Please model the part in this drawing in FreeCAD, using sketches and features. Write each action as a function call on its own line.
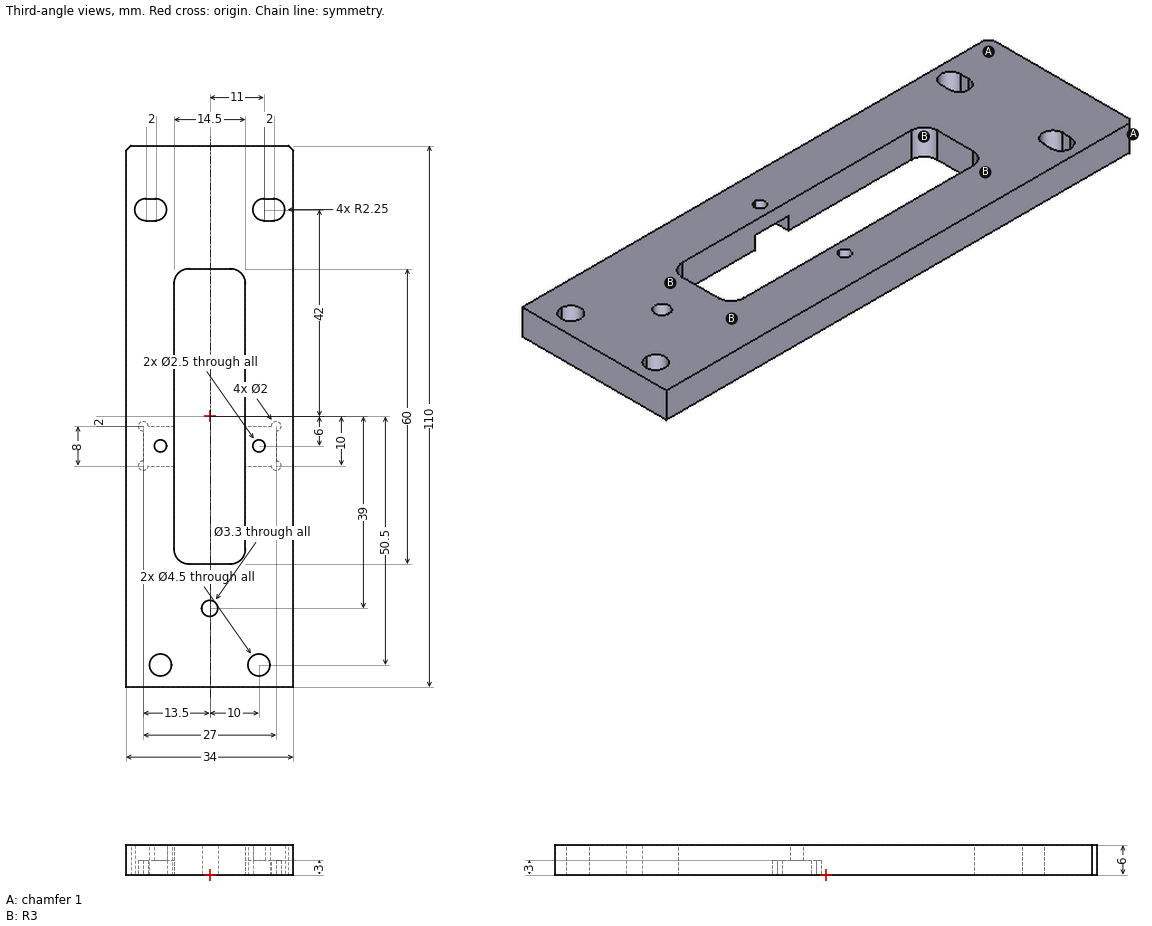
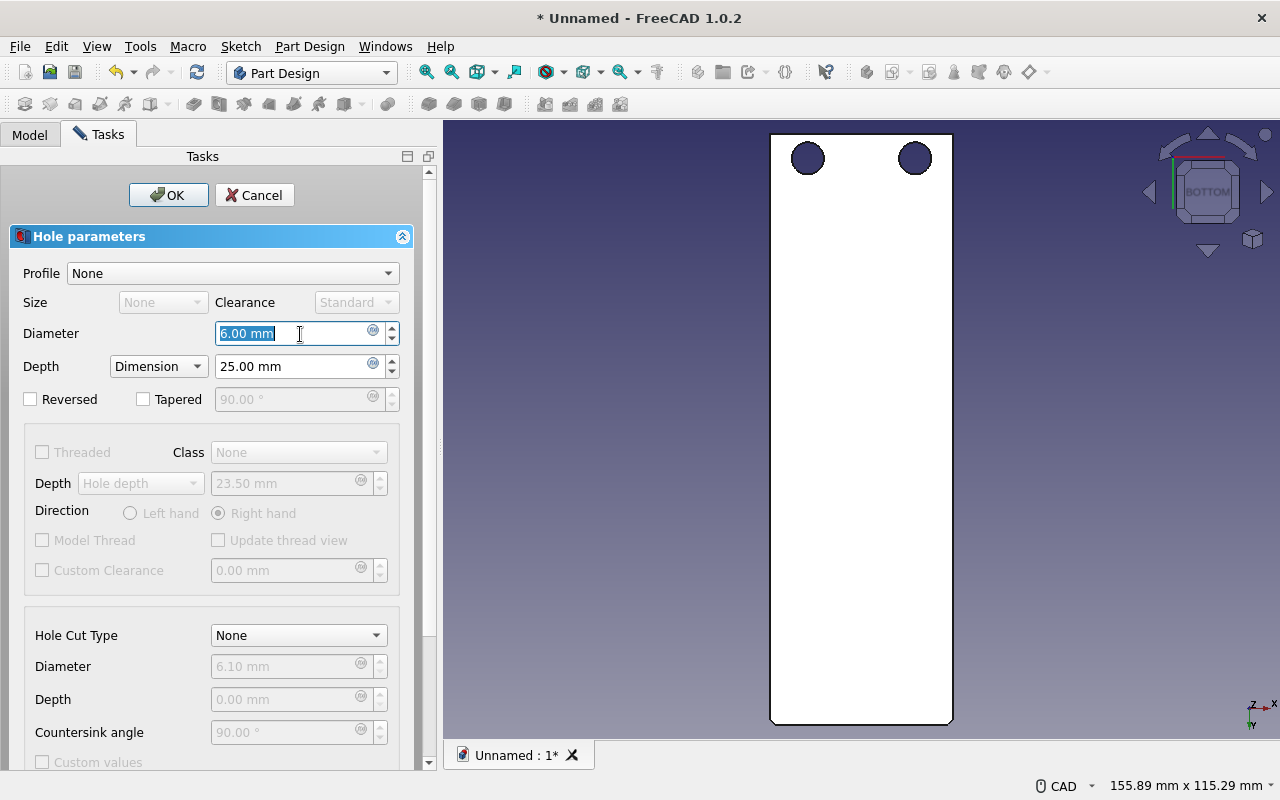
text(4.5)
key(Tab)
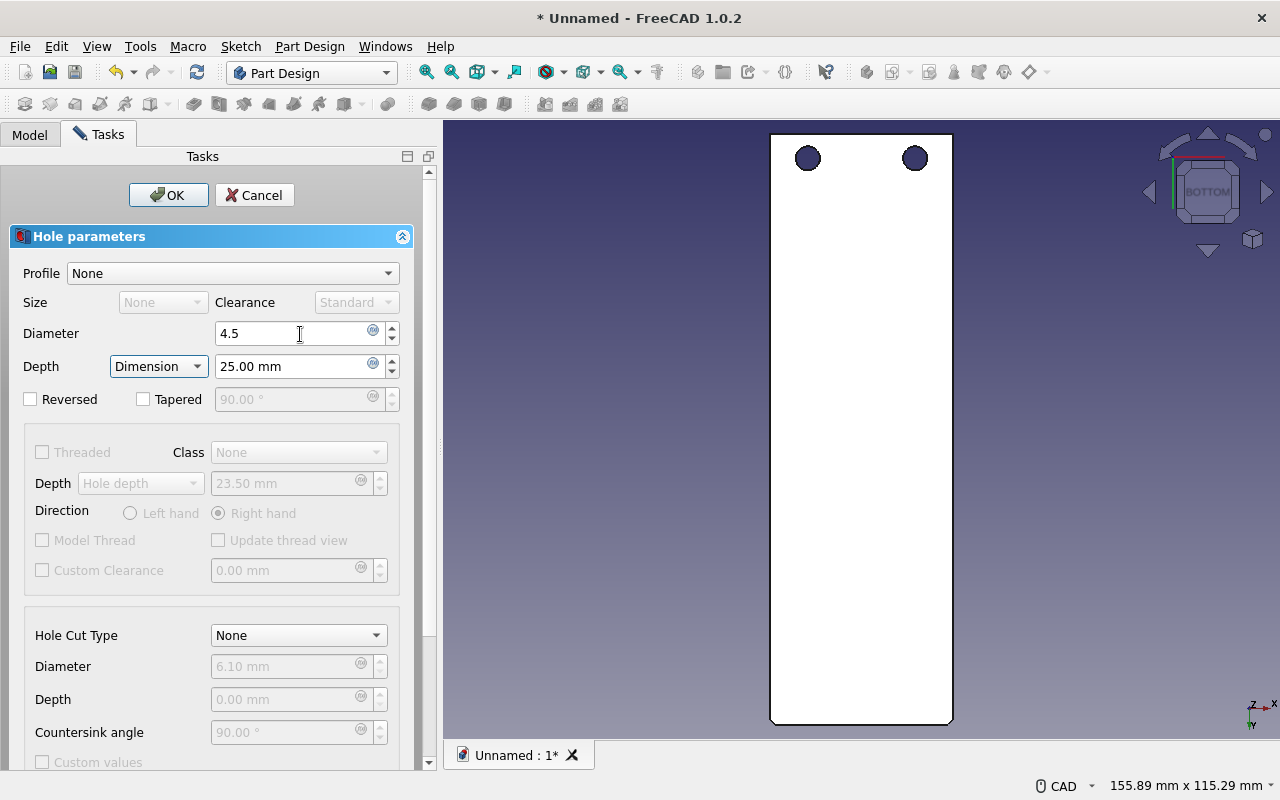
click(160, 366)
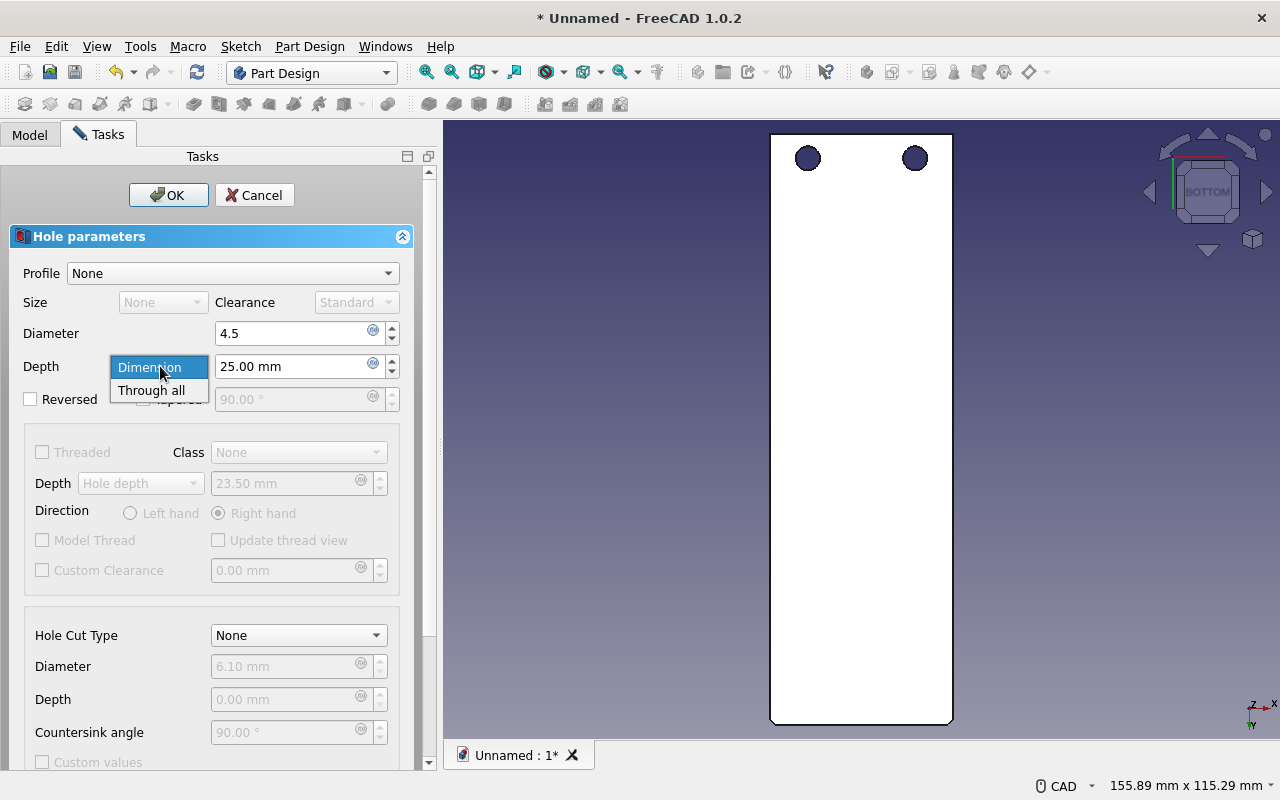
click(158, 390)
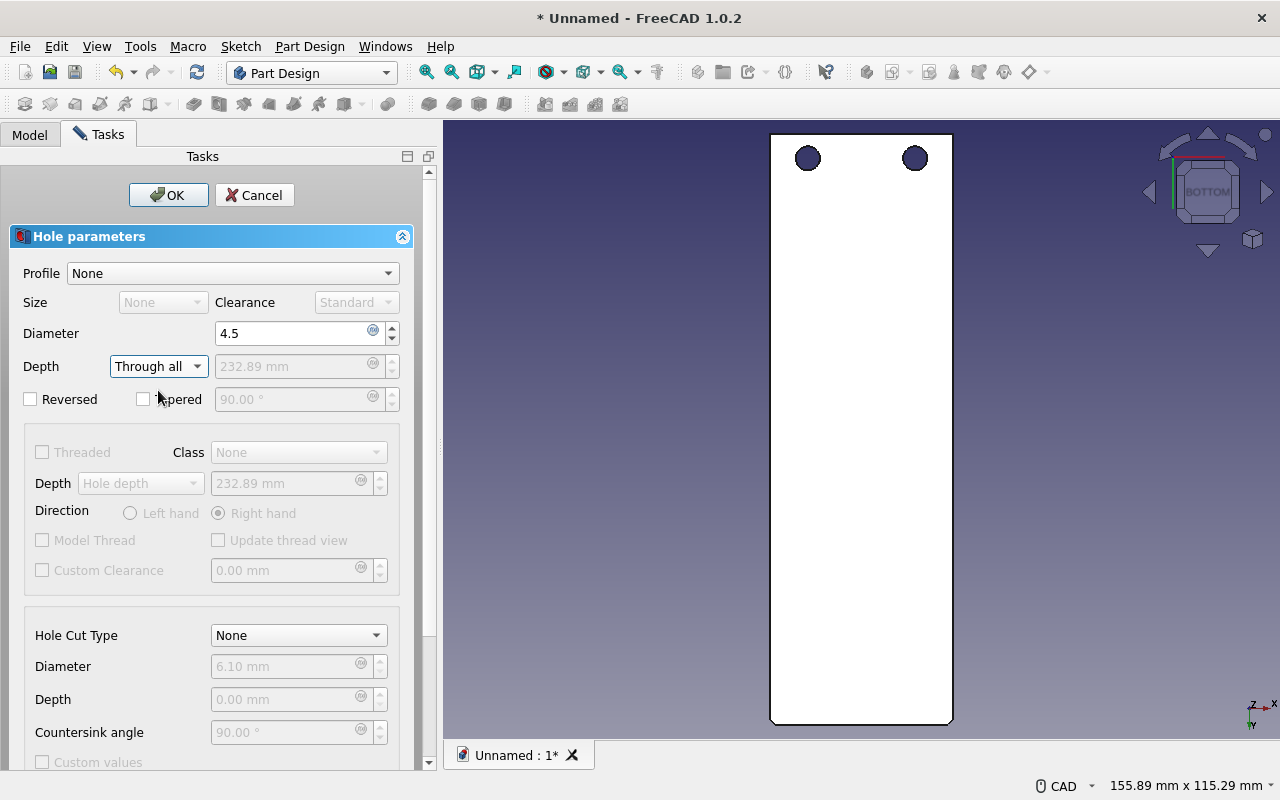
click(169, 195)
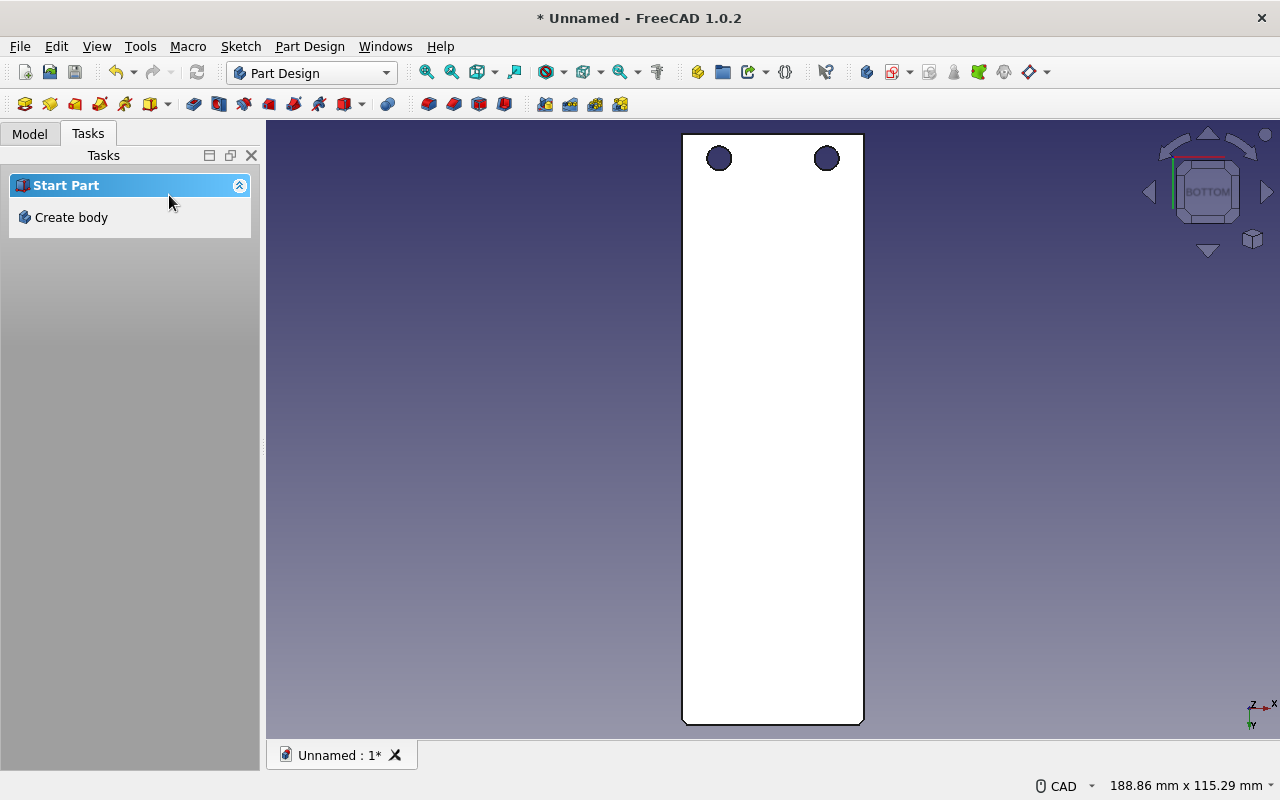
click(773, 597)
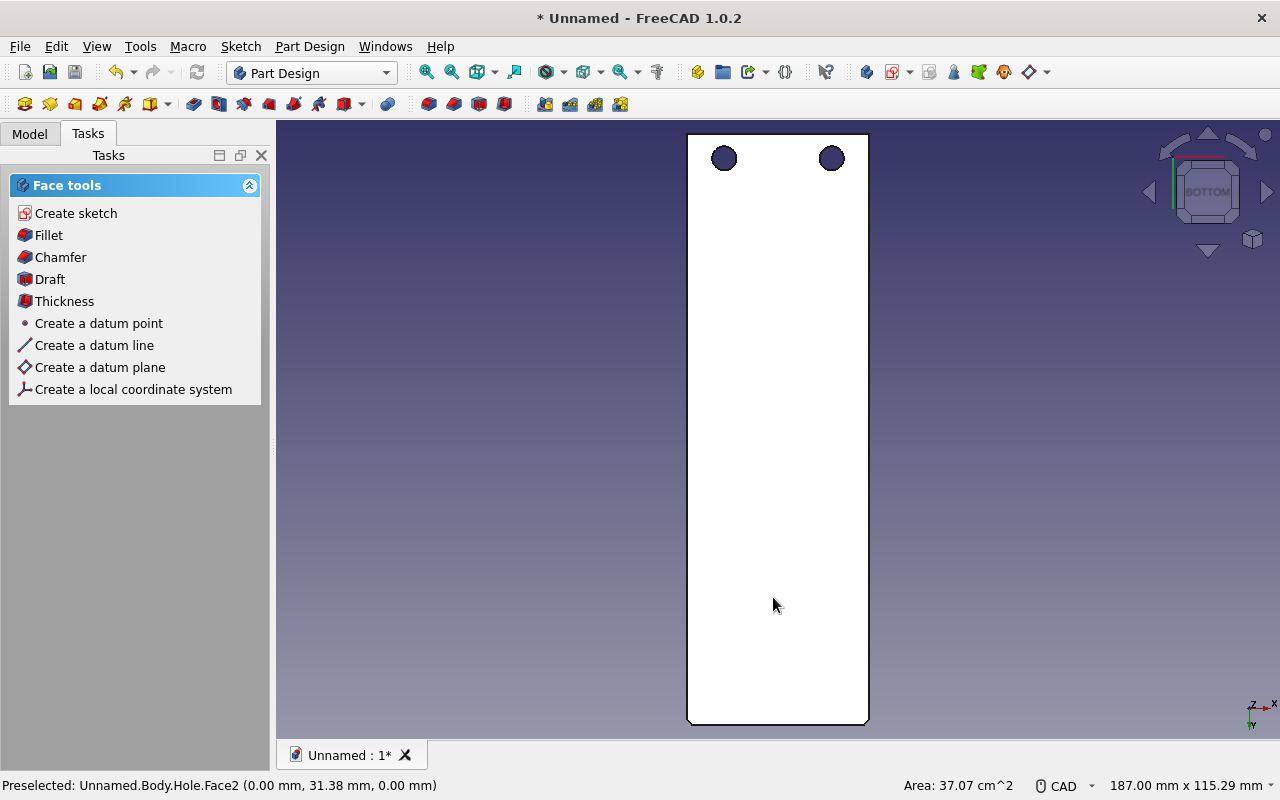
click(892, 72)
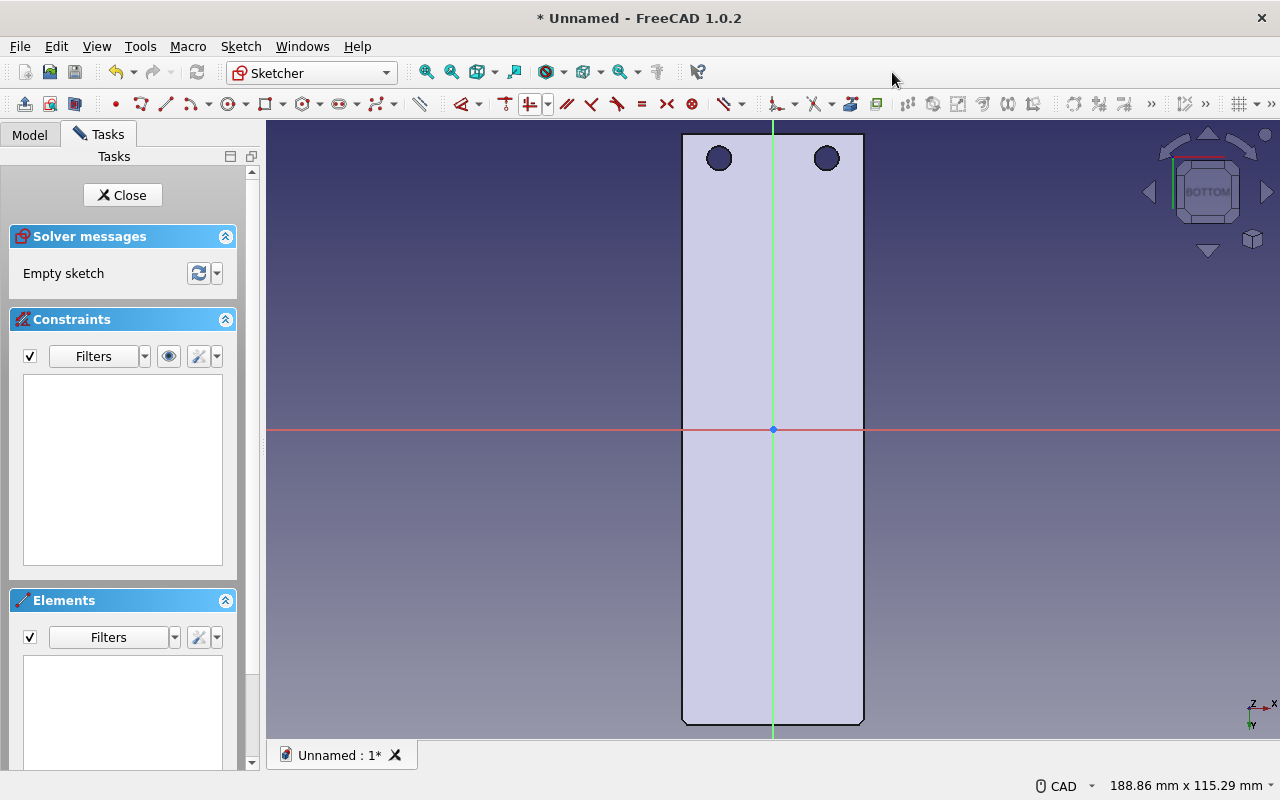
scroll(856, 693, up, 3)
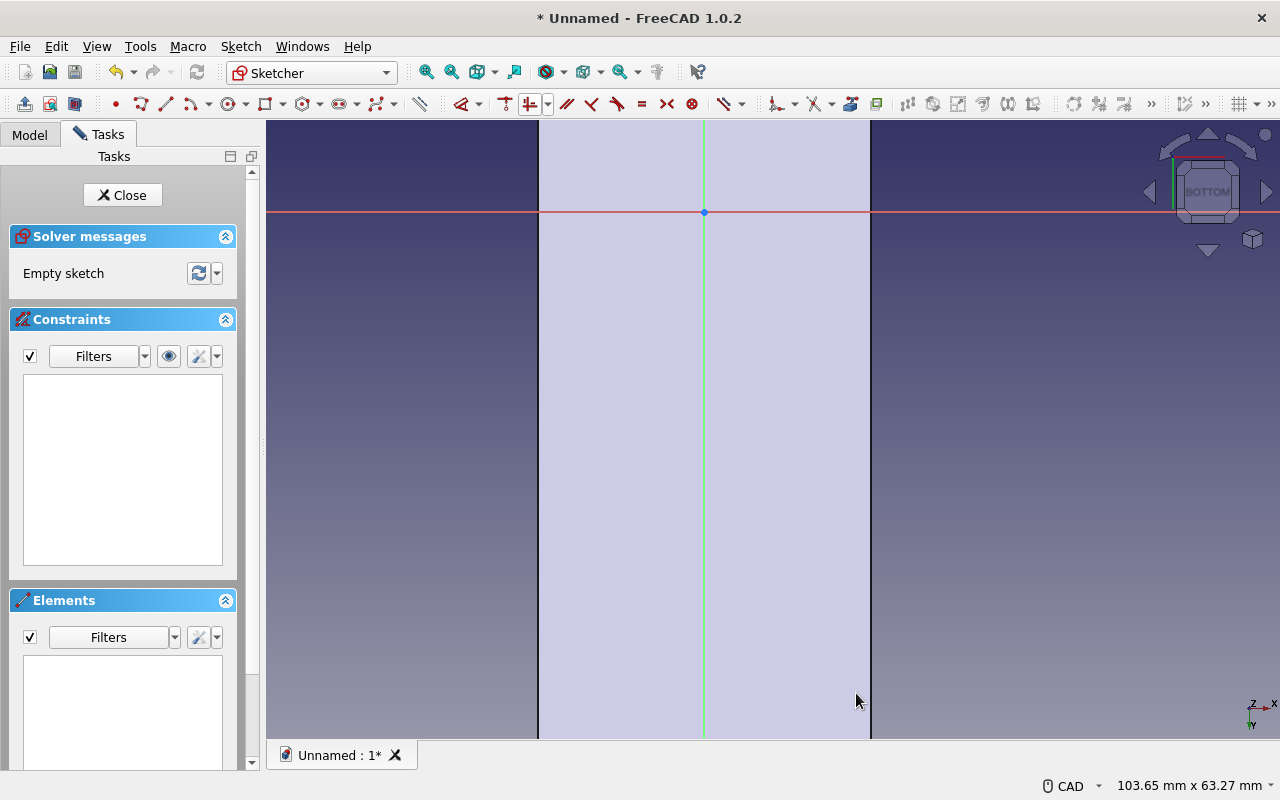
key(g)
key(s)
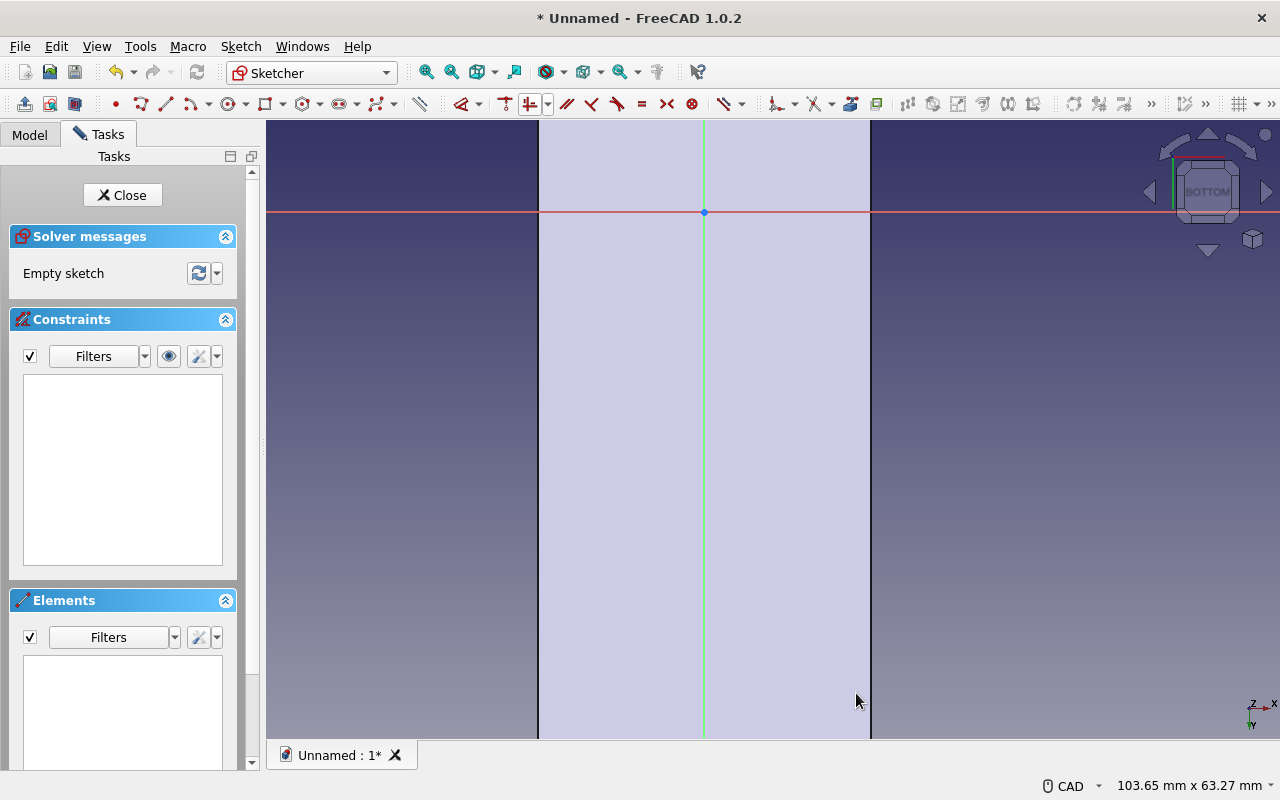
click(812, 623)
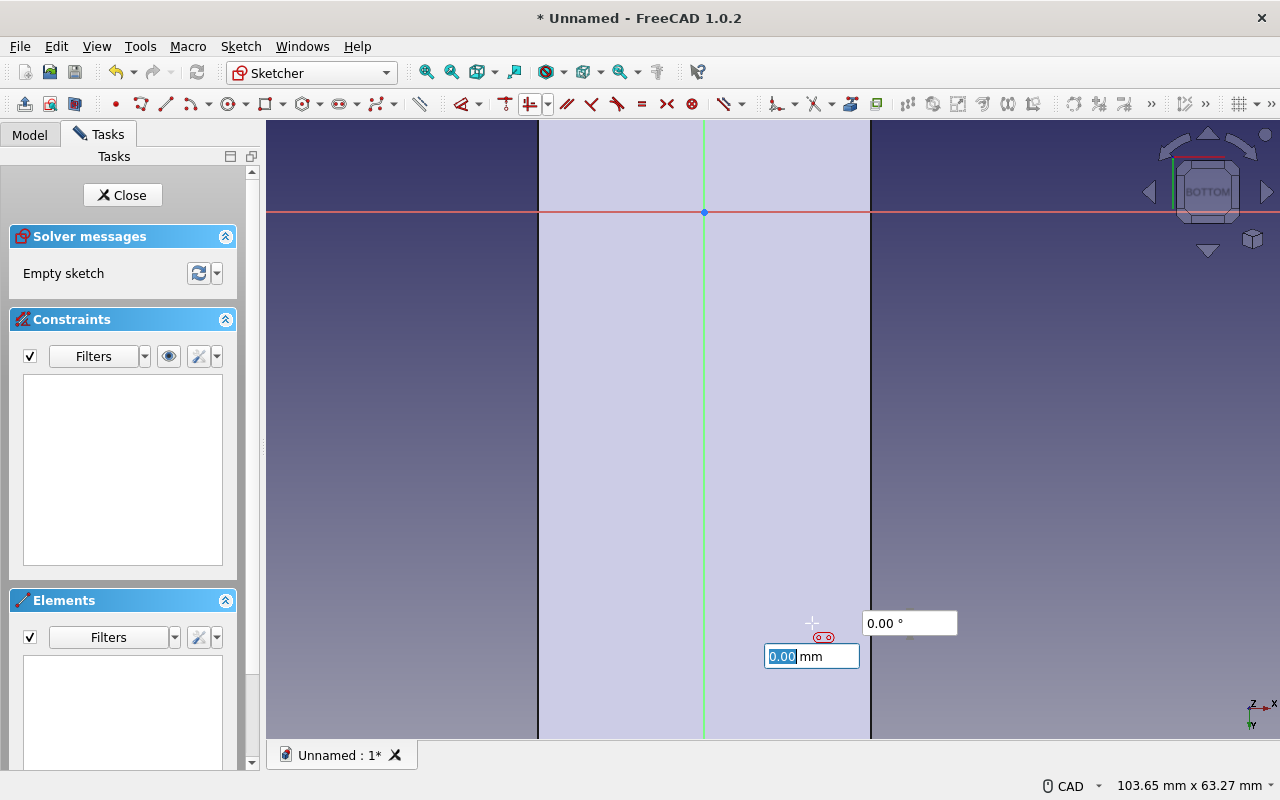
click(831, 623)